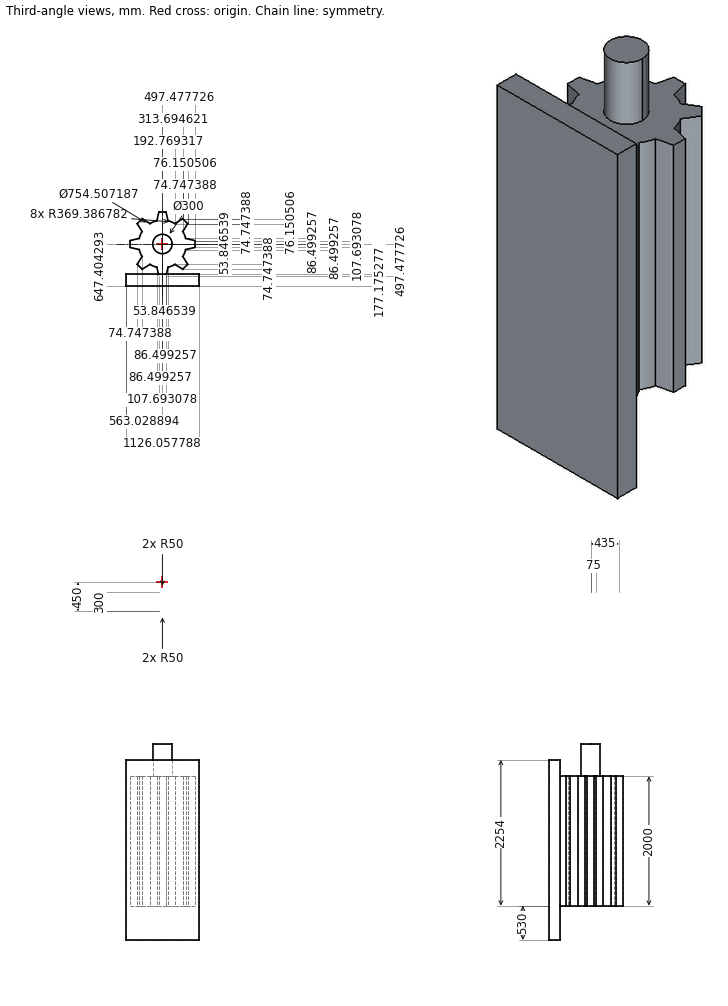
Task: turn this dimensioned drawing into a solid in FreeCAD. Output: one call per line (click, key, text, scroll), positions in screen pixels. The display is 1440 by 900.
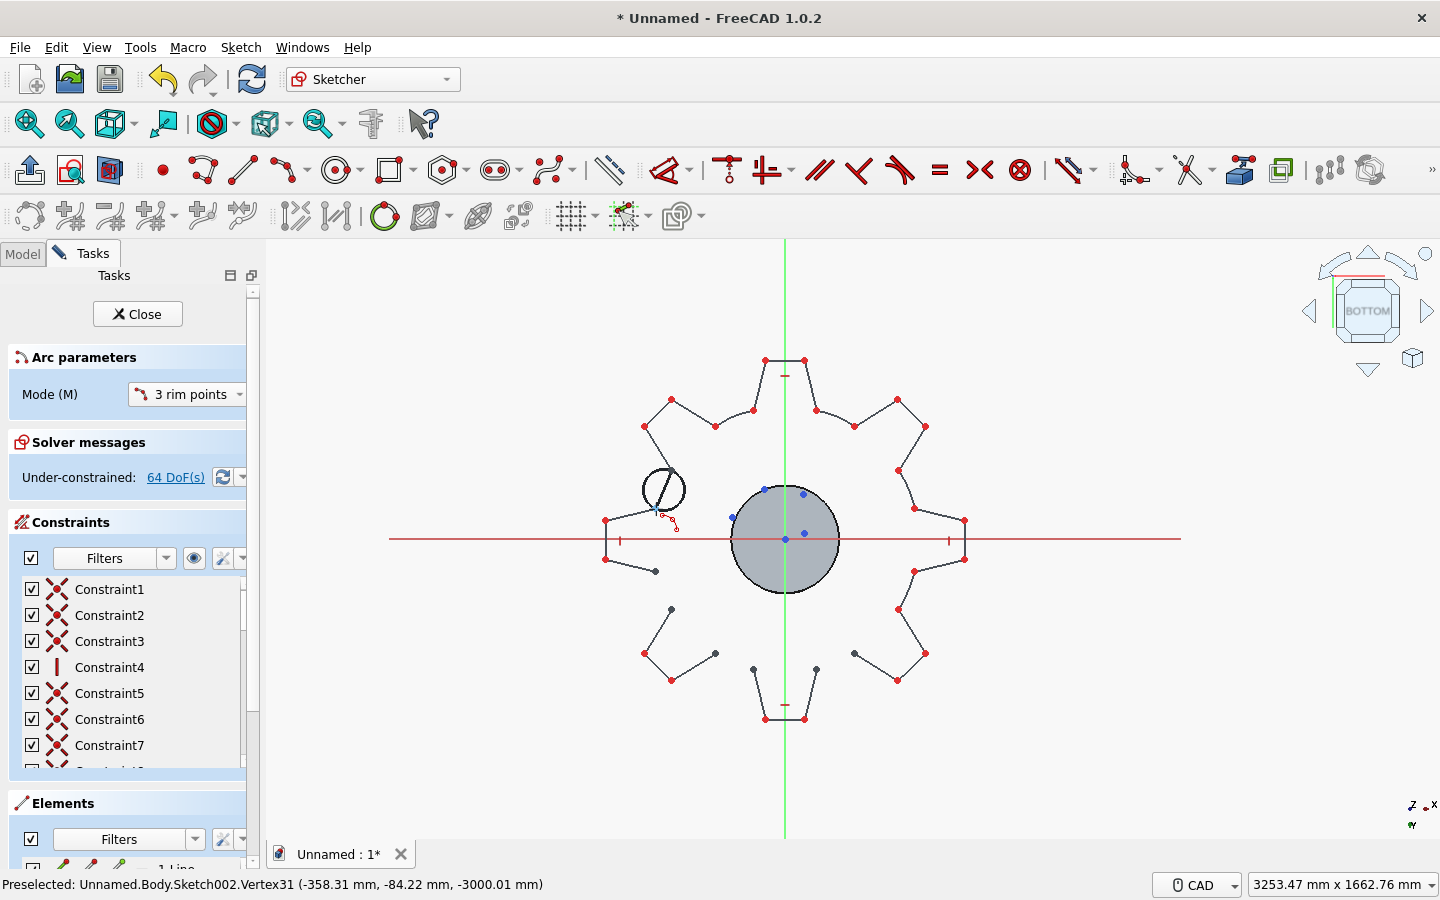
scroll(662, 488, up, 12)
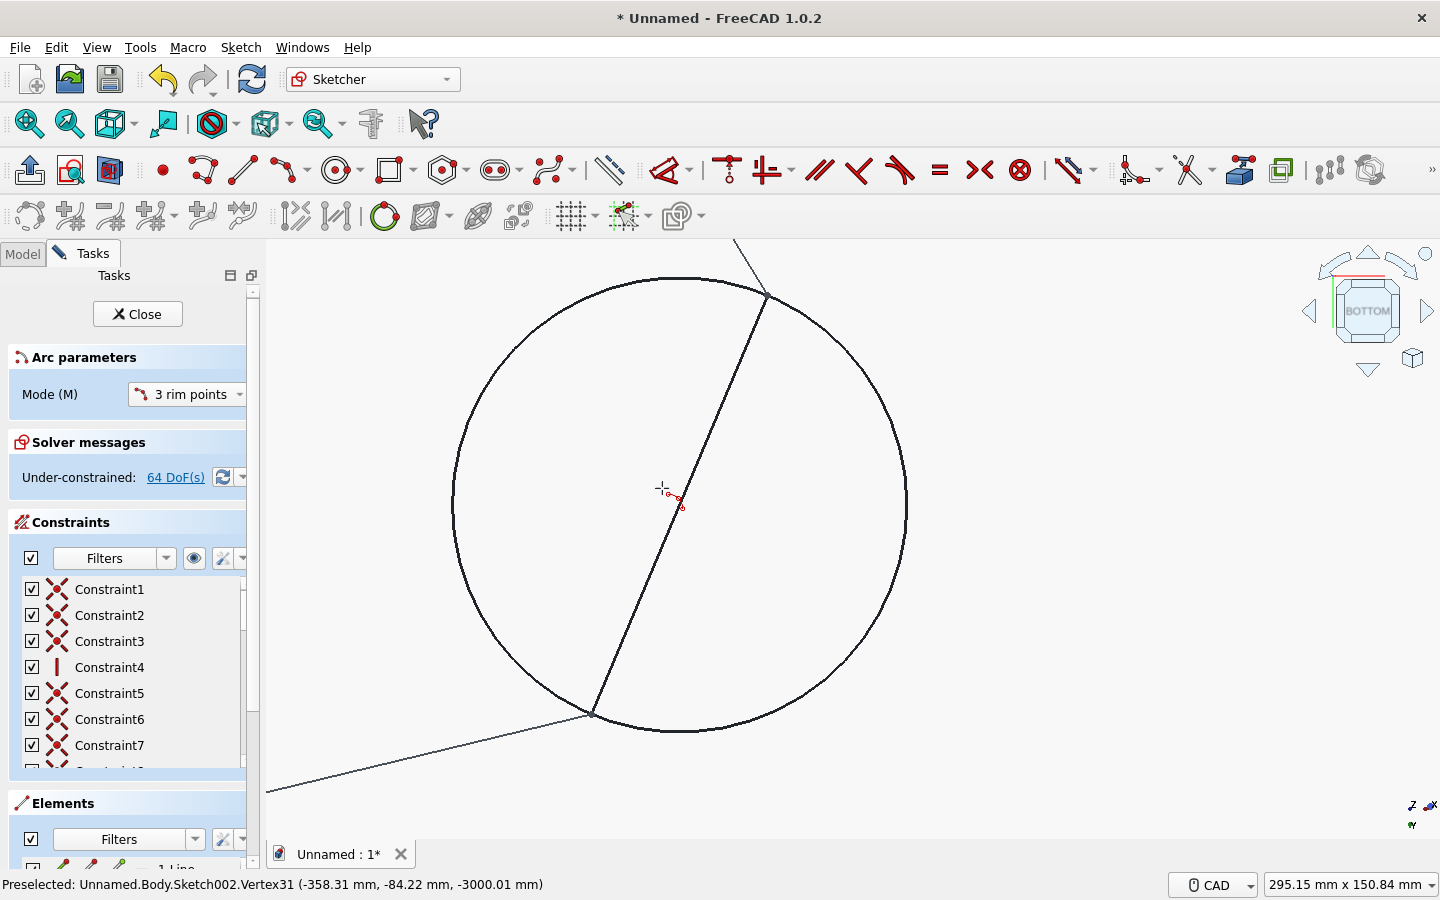
click(659, 487)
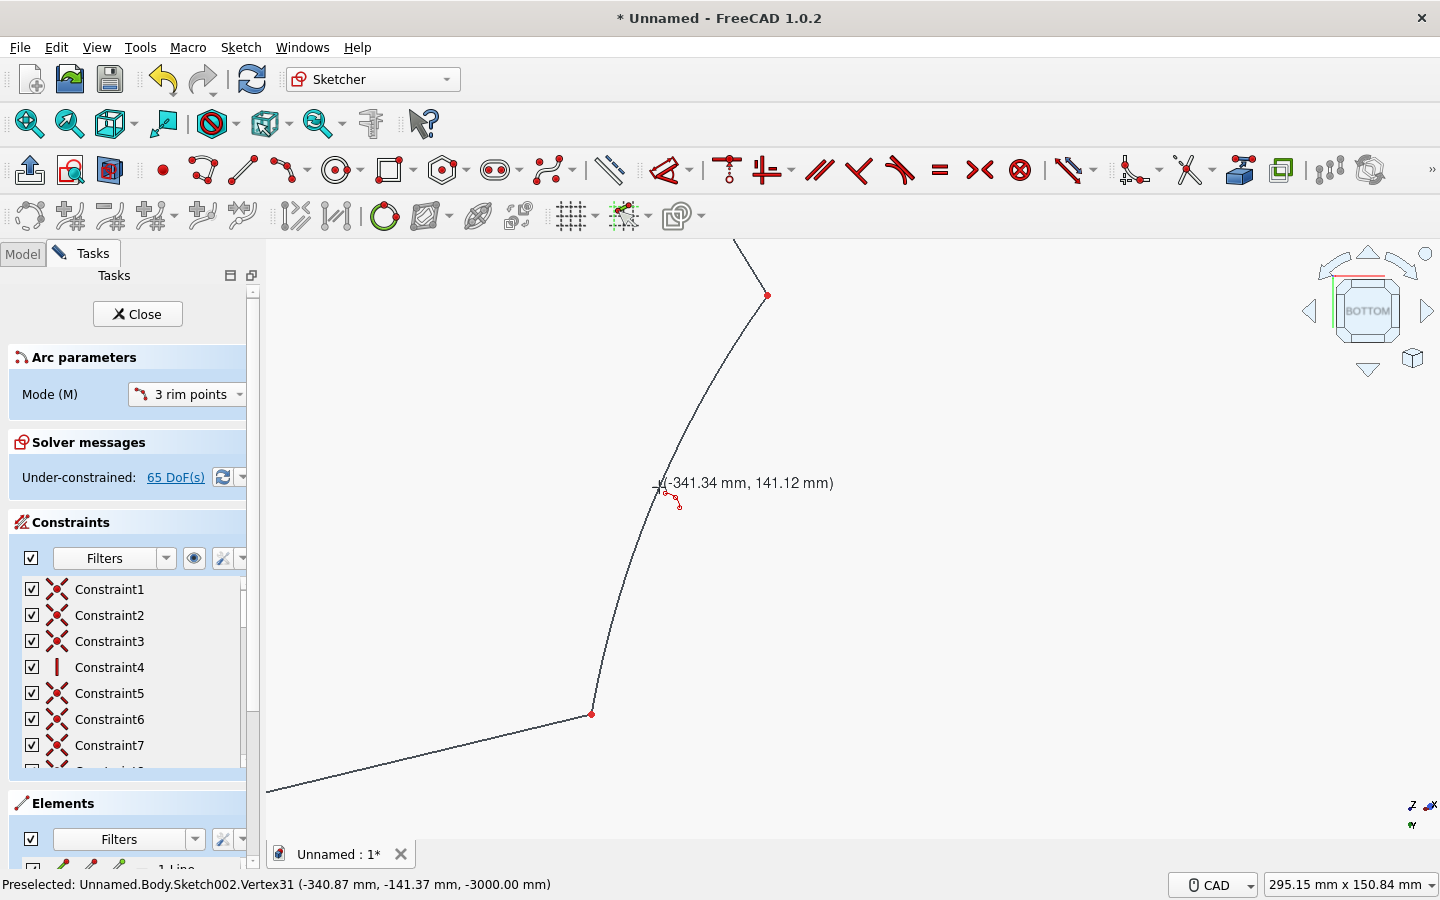
scroll(662, 488, down, 12)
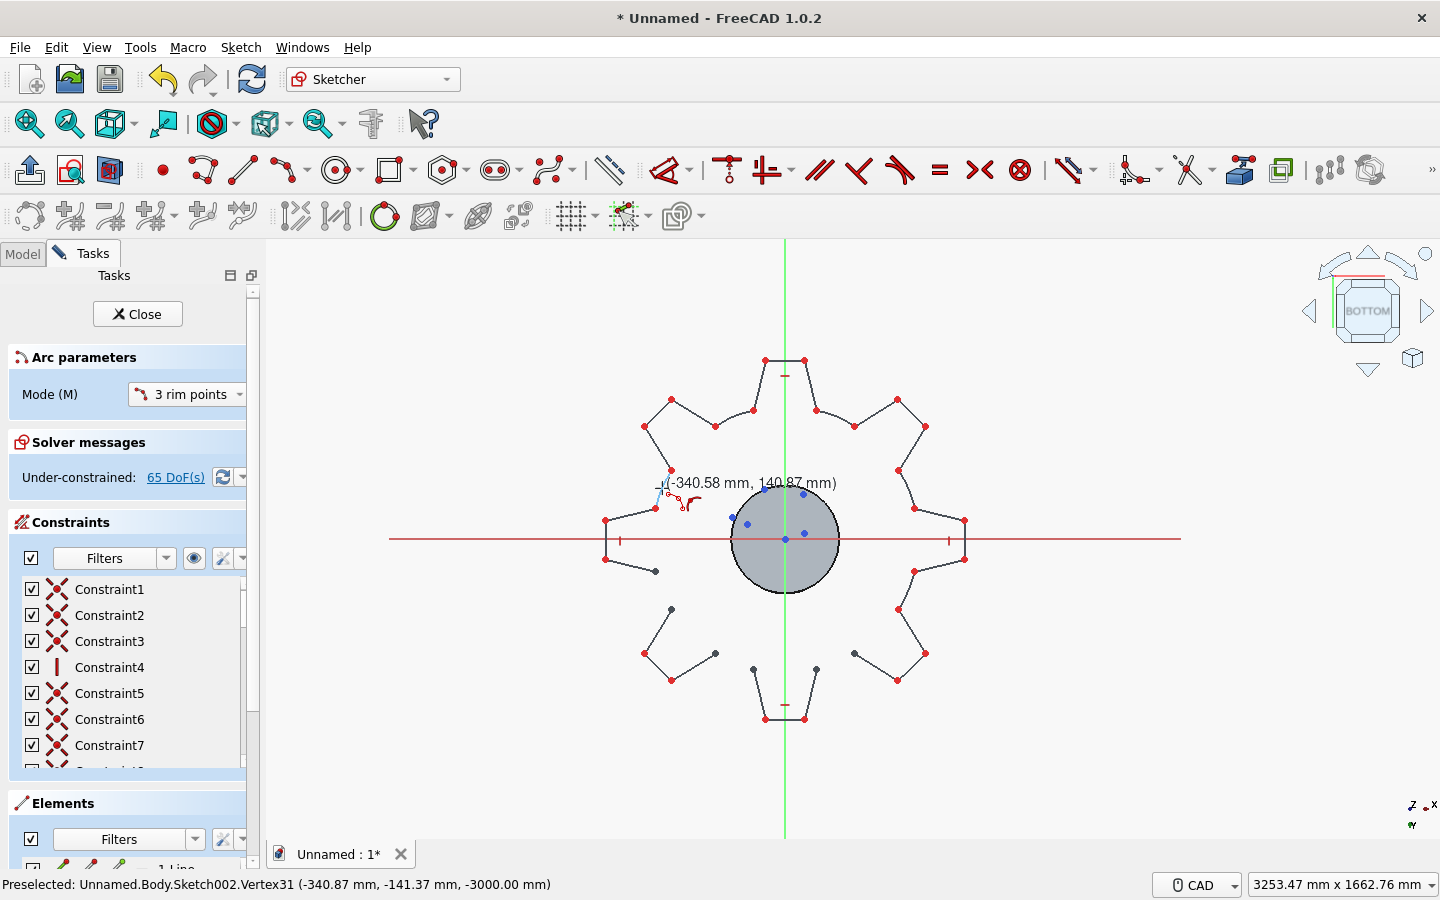
click(656, 572)
click(672, 610)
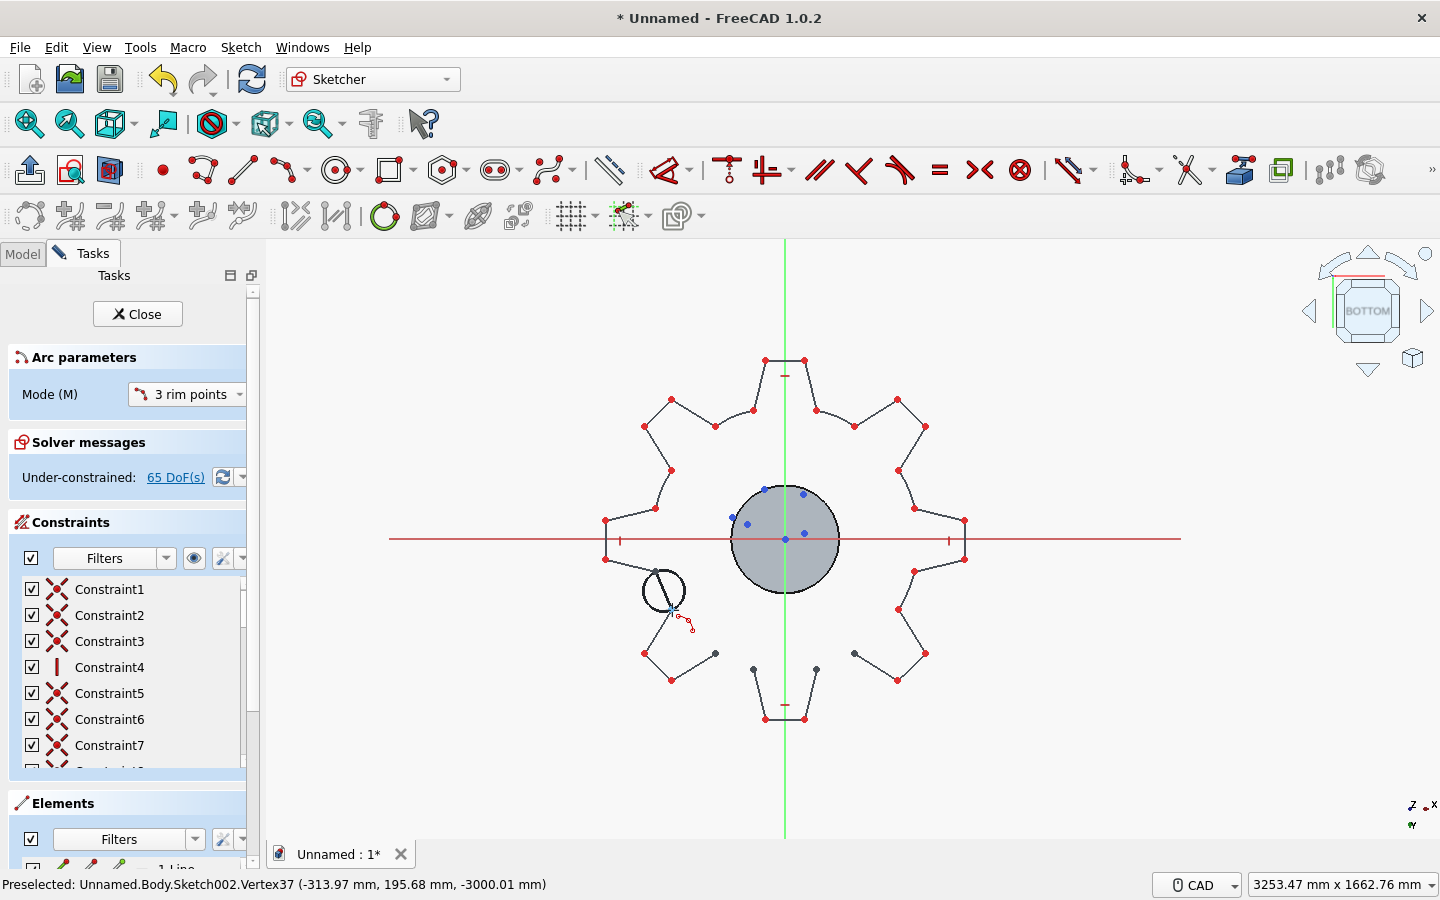
scroll(662, 590, up, 12)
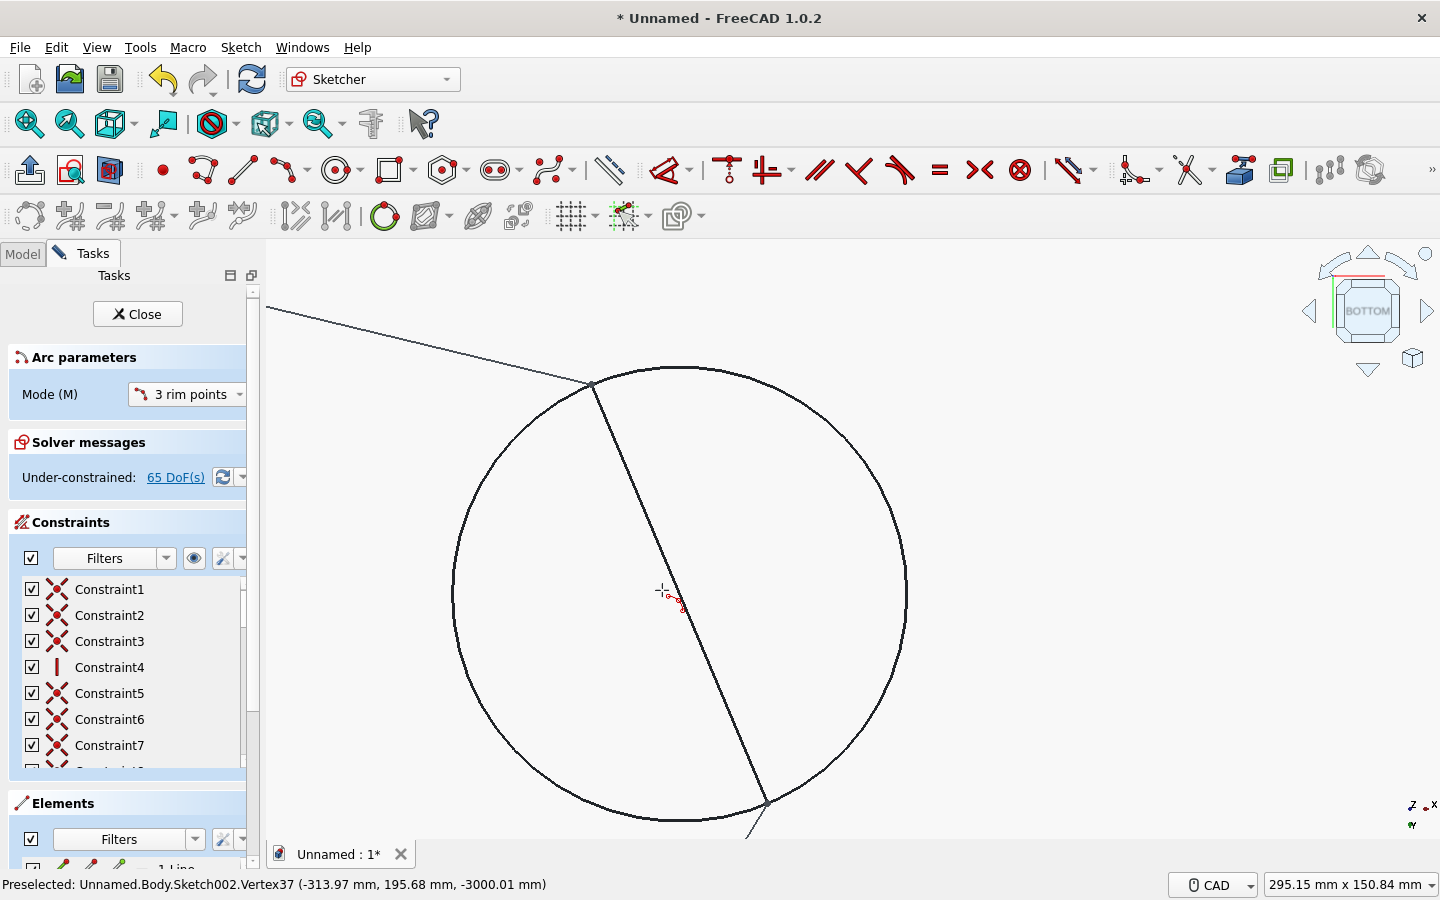
click(659, 588)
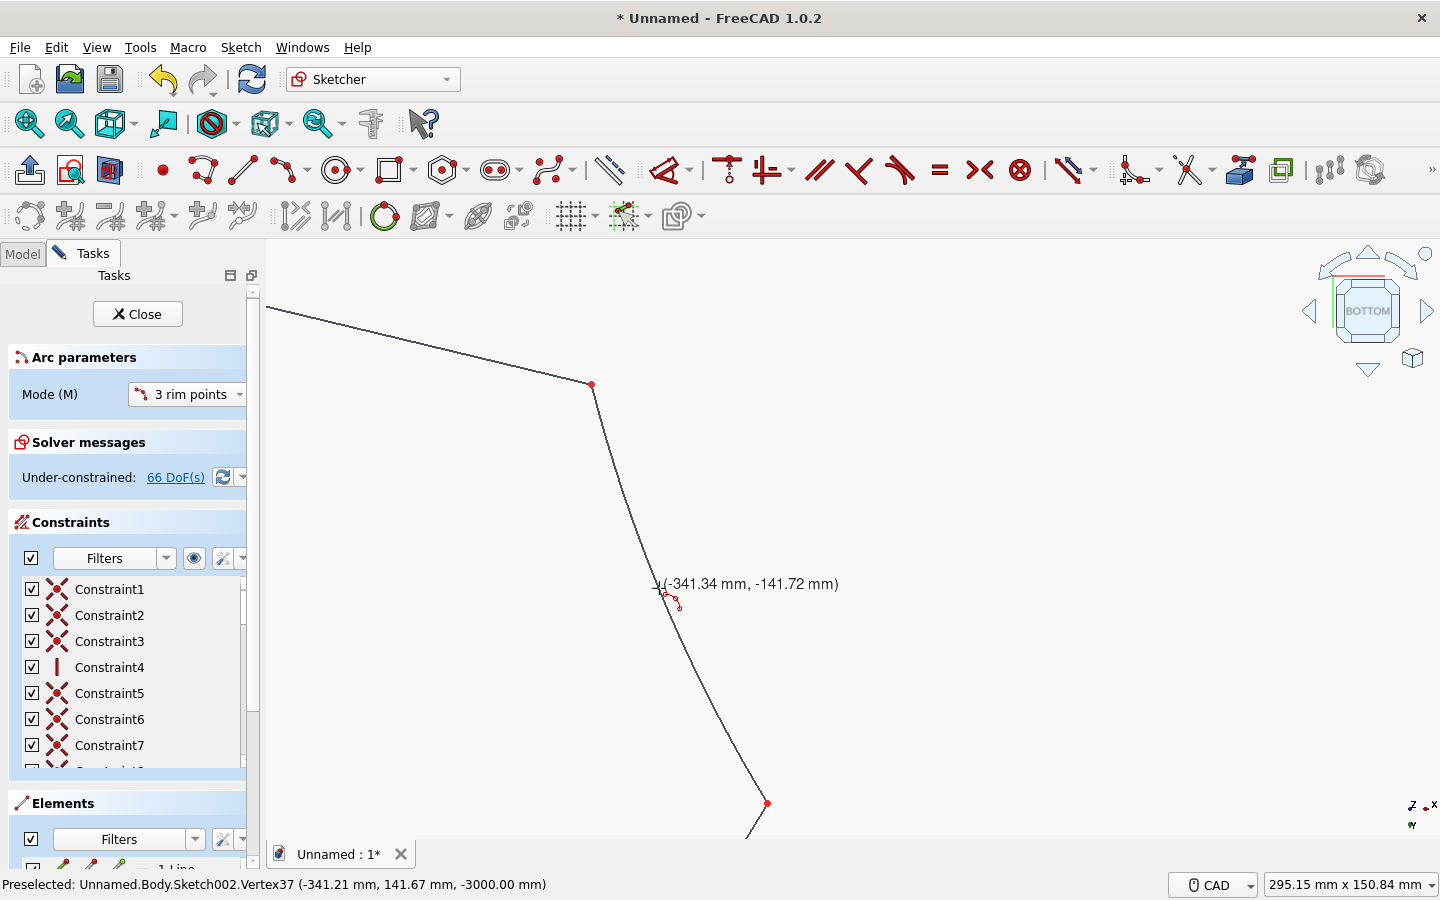
scroll(662, 590, down, 12)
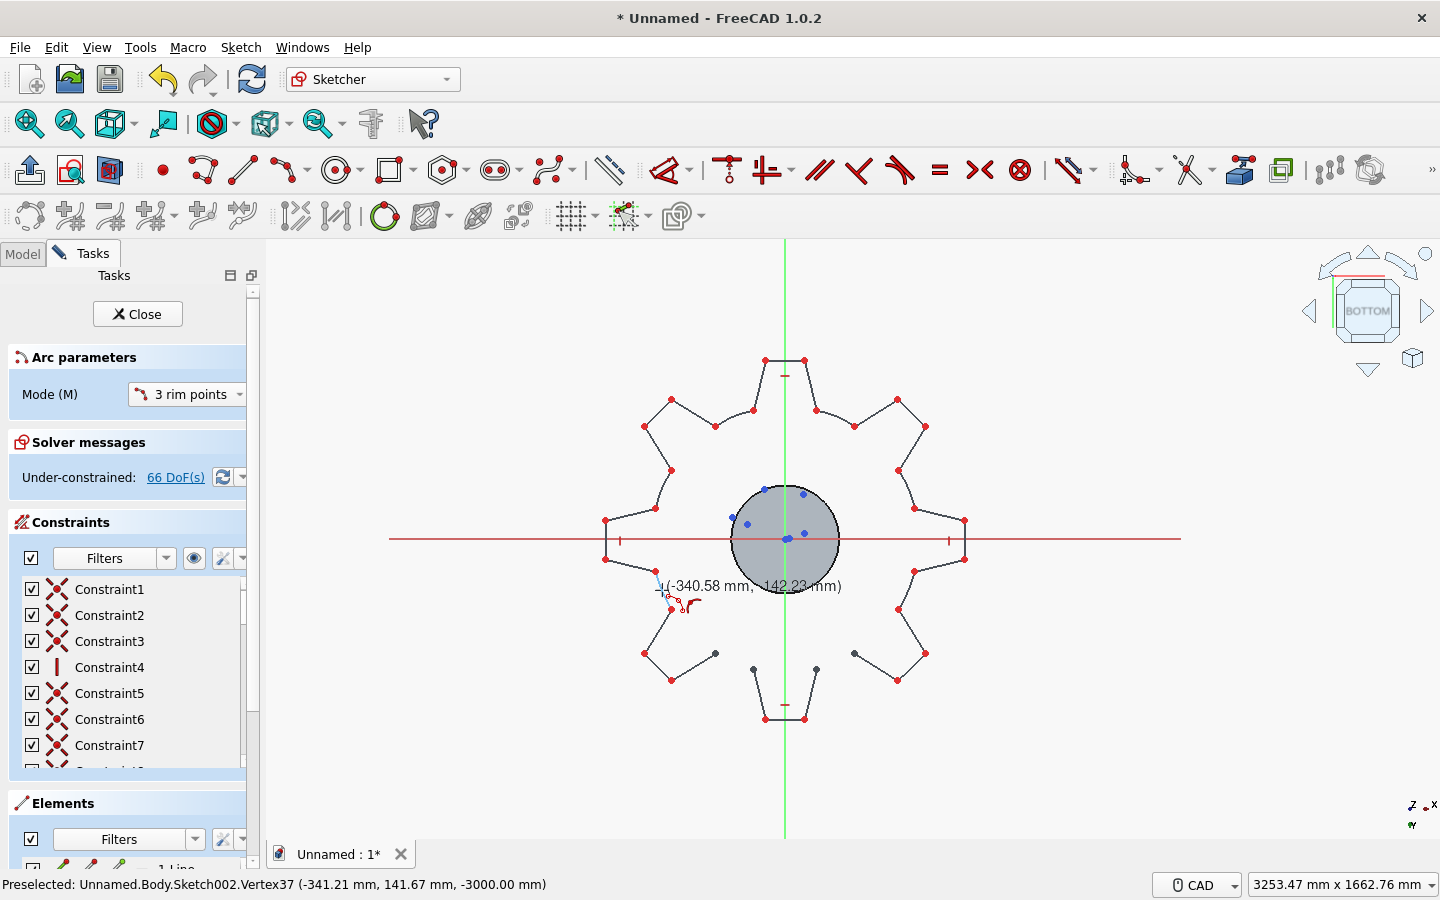
click(716, 654)
click(754, 670)